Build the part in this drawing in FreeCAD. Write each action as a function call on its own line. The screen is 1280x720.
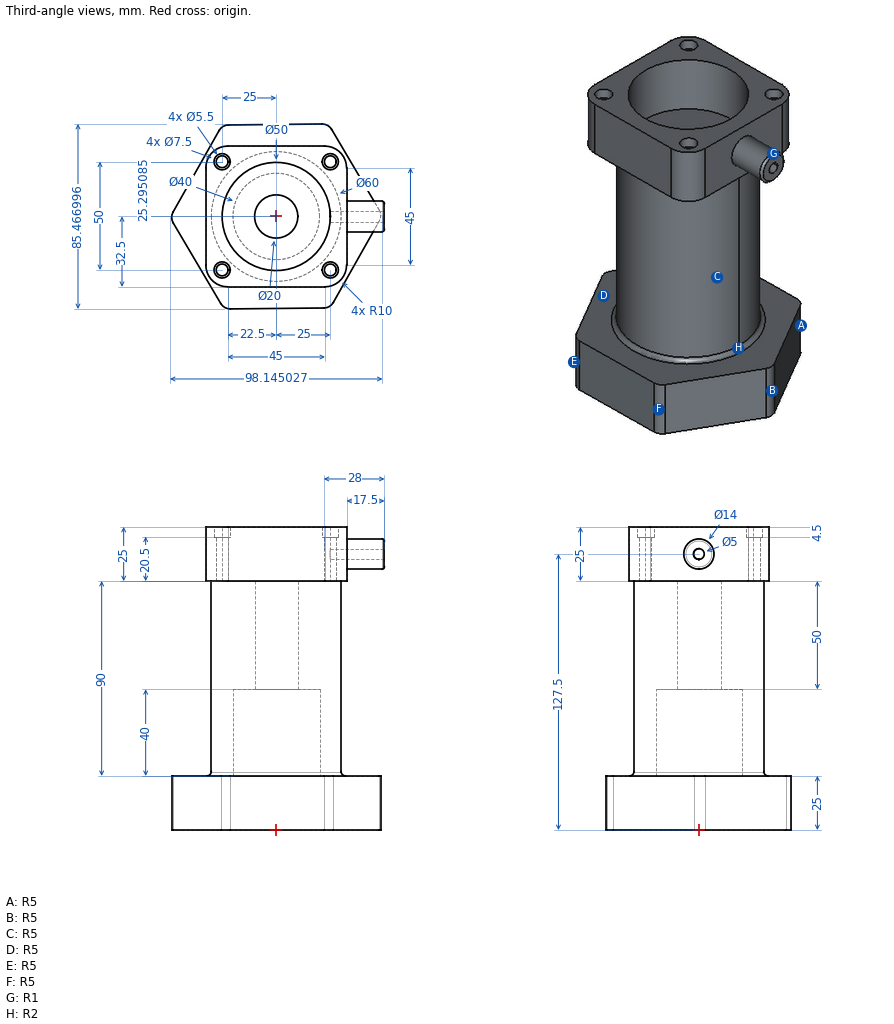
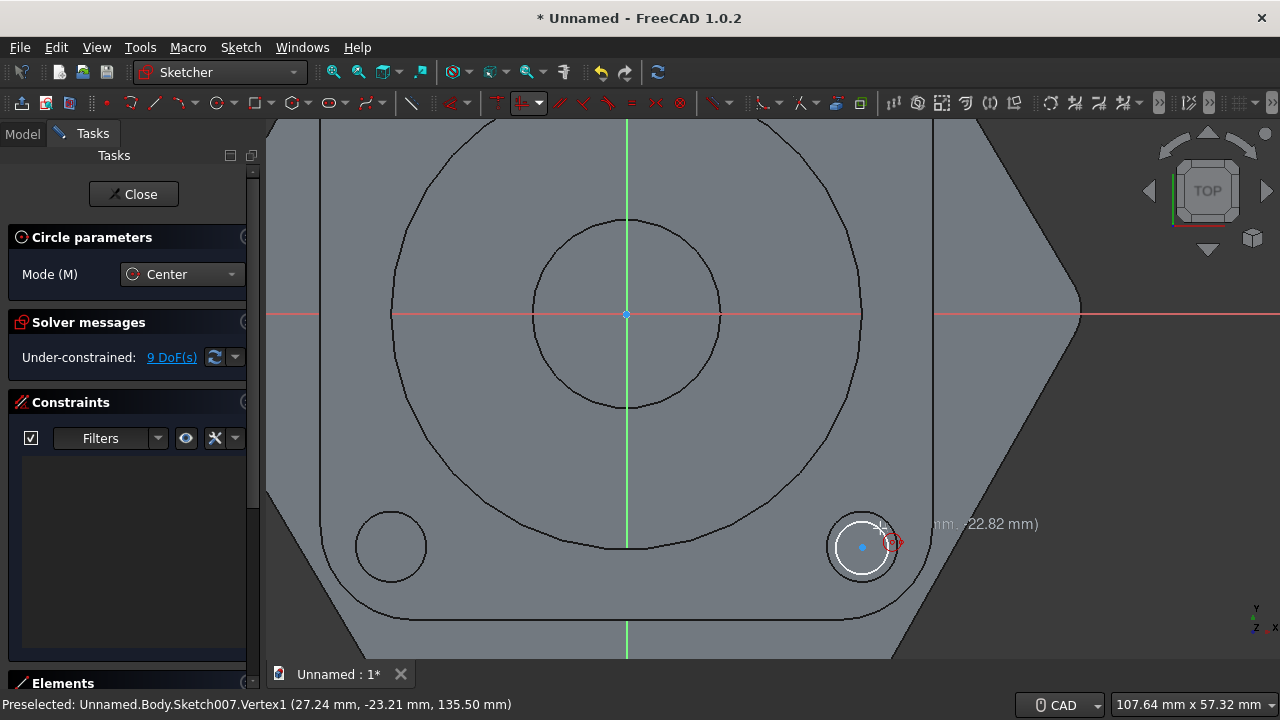
click(391, 547)
click(409, 528)
key(Escape)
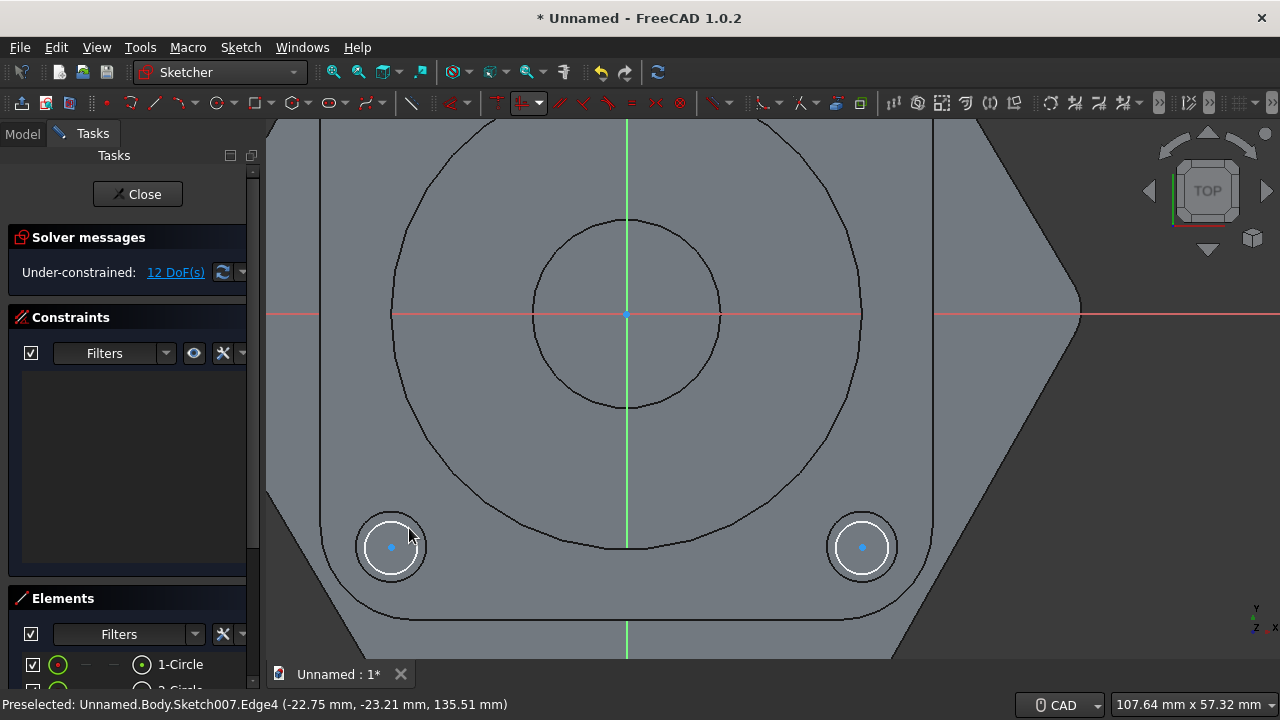
scroll(863, 547, down, 2)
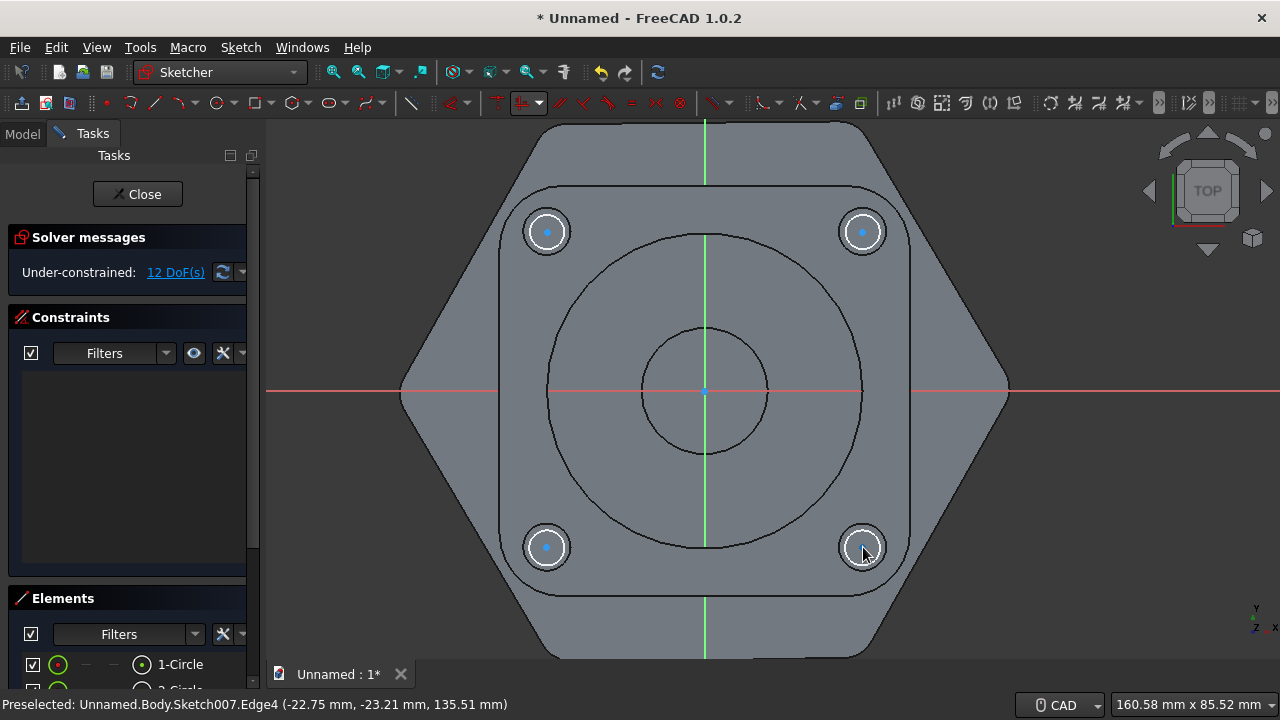
click(559, 220)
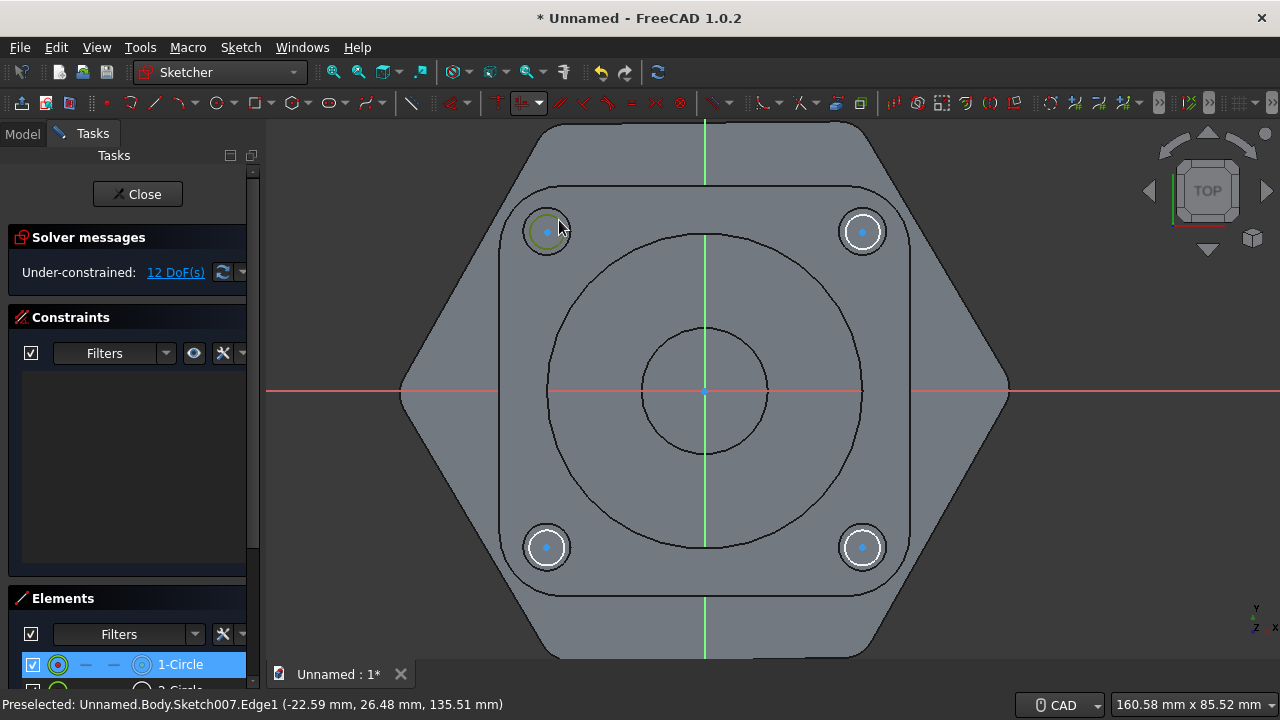
click(875, 220)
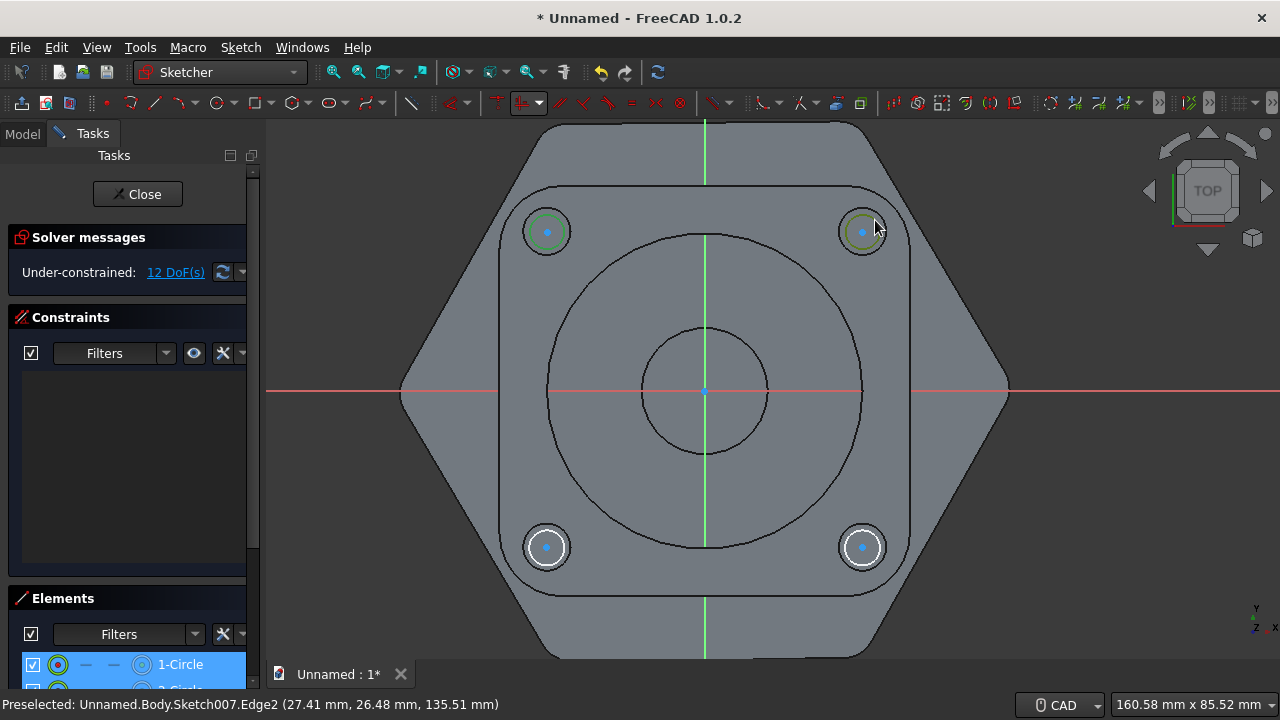
click(875, 535)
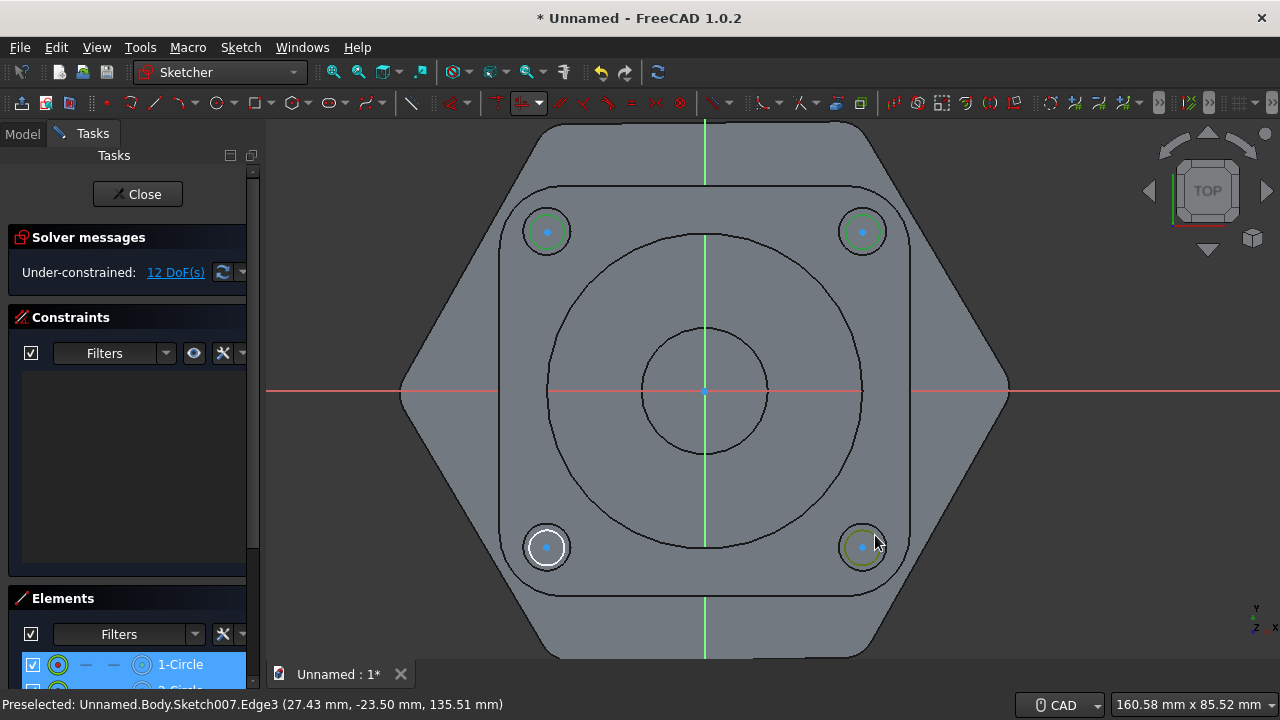
click(559, 535)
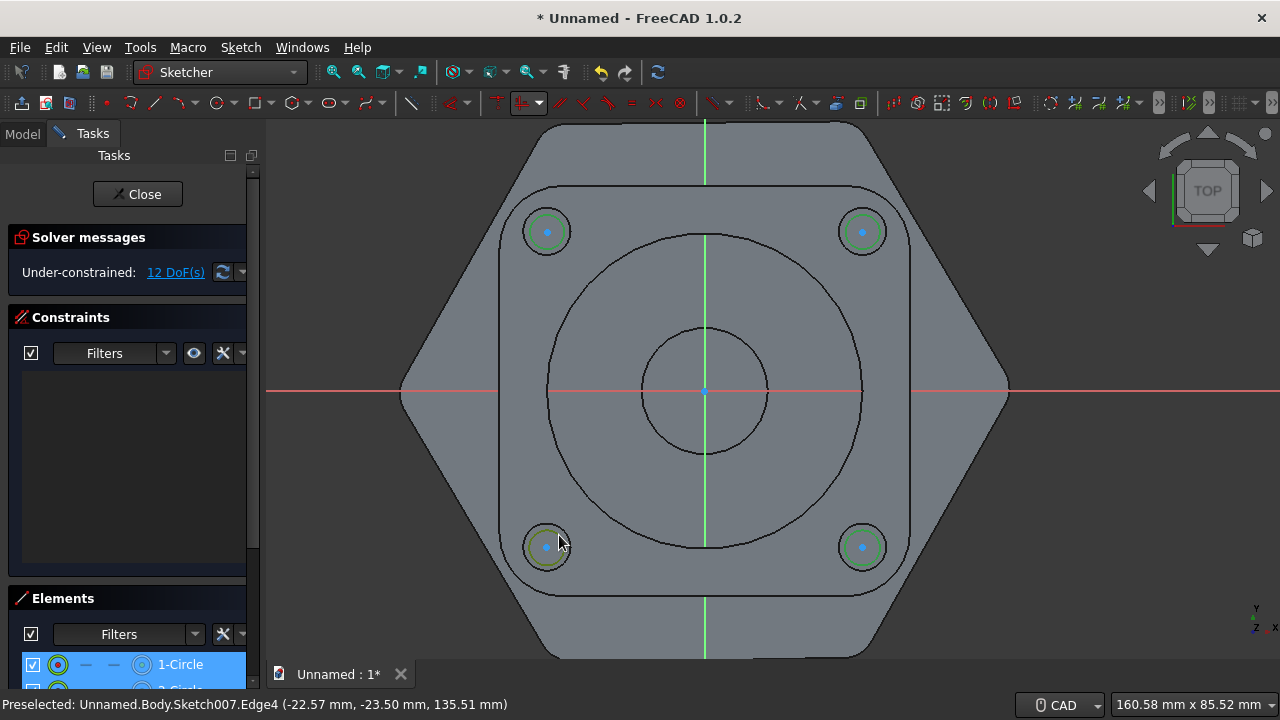
click(632, 104)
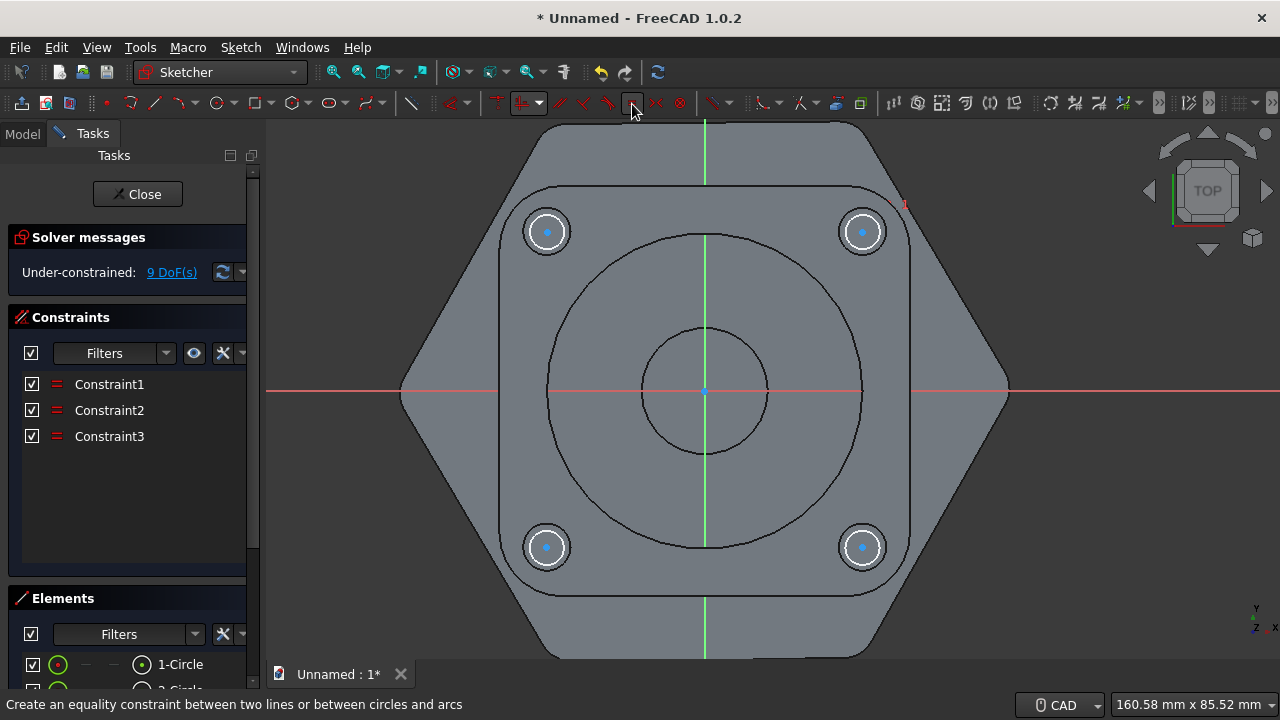
click(547, 232)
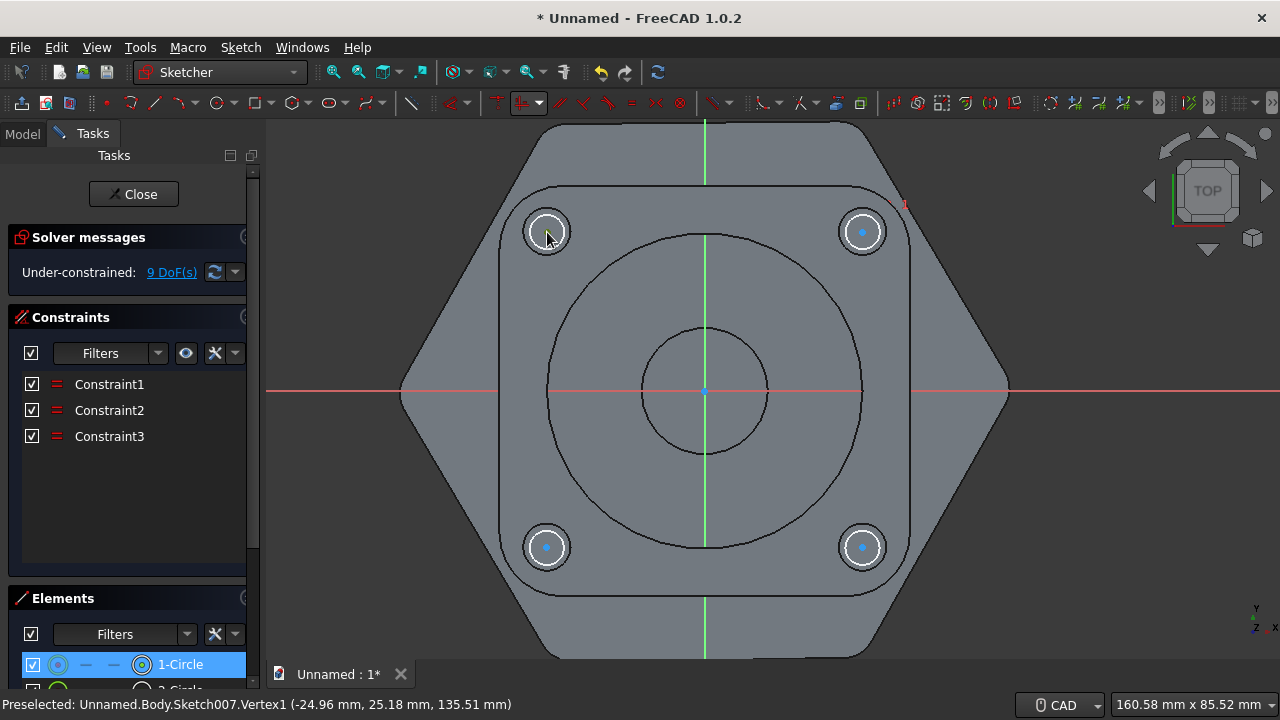
click(863, 232)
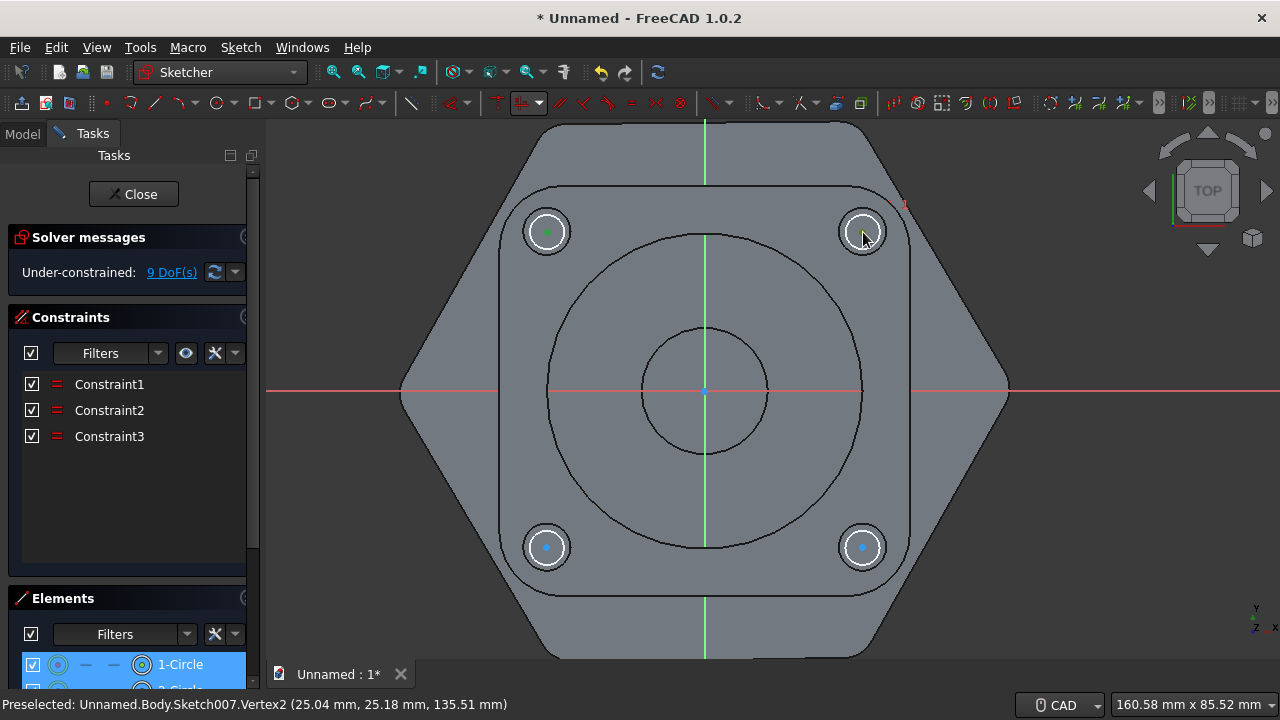
click(542, 104)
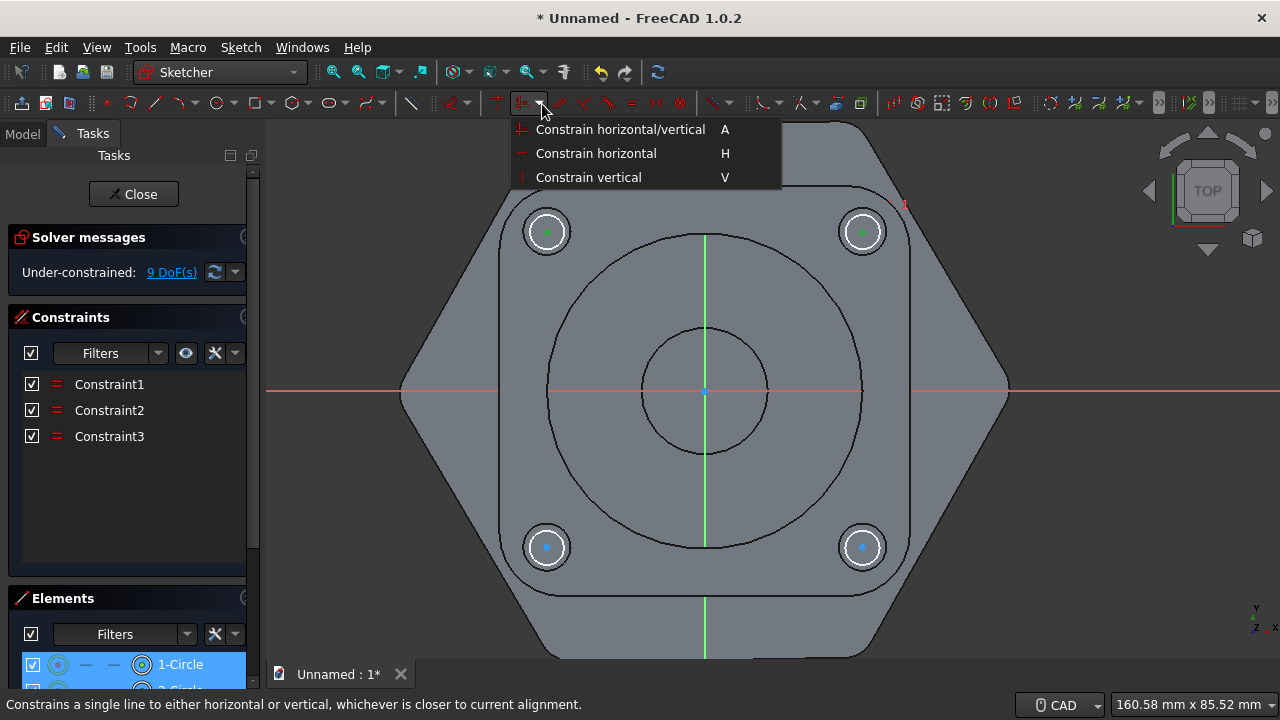
click(646, 153)